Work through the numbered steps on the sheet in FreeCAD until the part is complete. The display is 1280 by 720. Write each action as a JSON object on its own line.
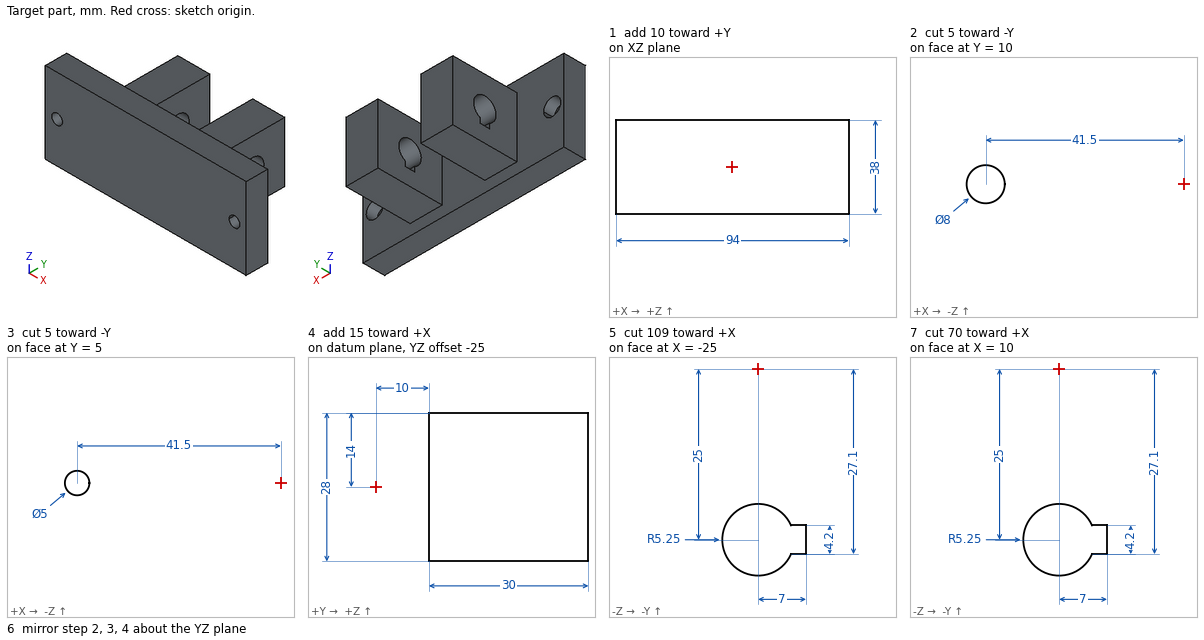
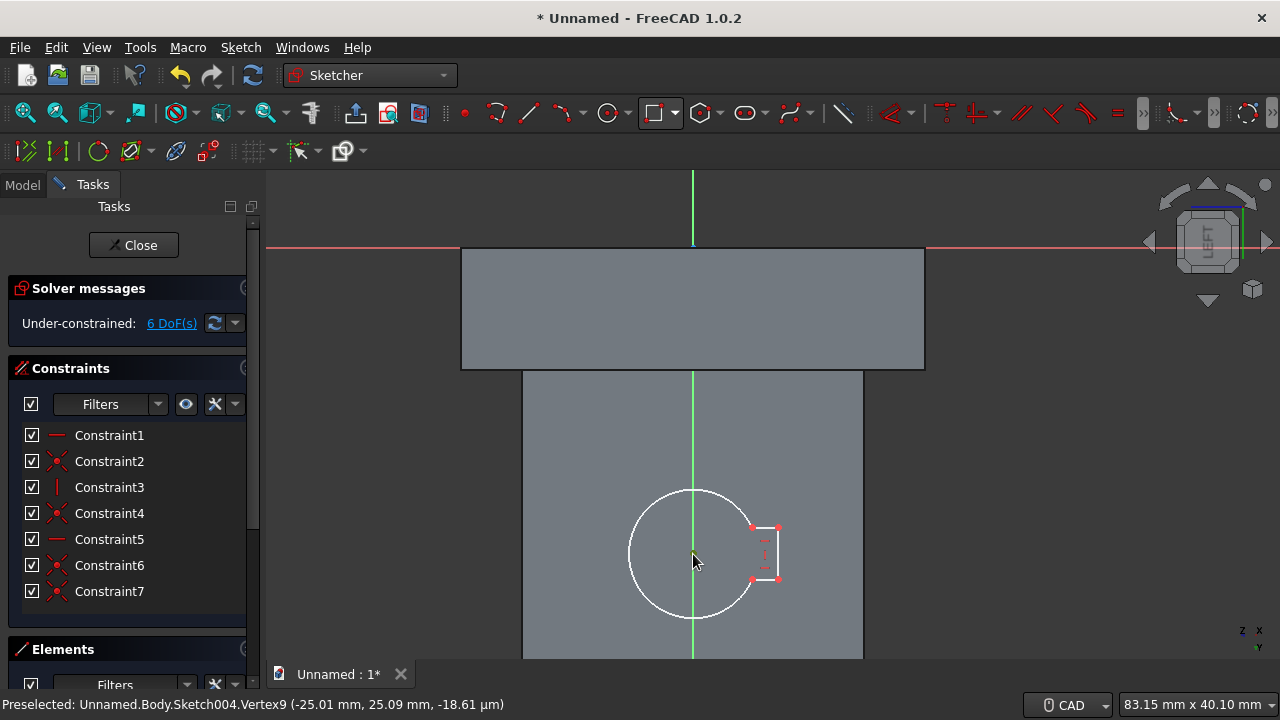
{"action": "left_click", "coordinate": [693, 569]}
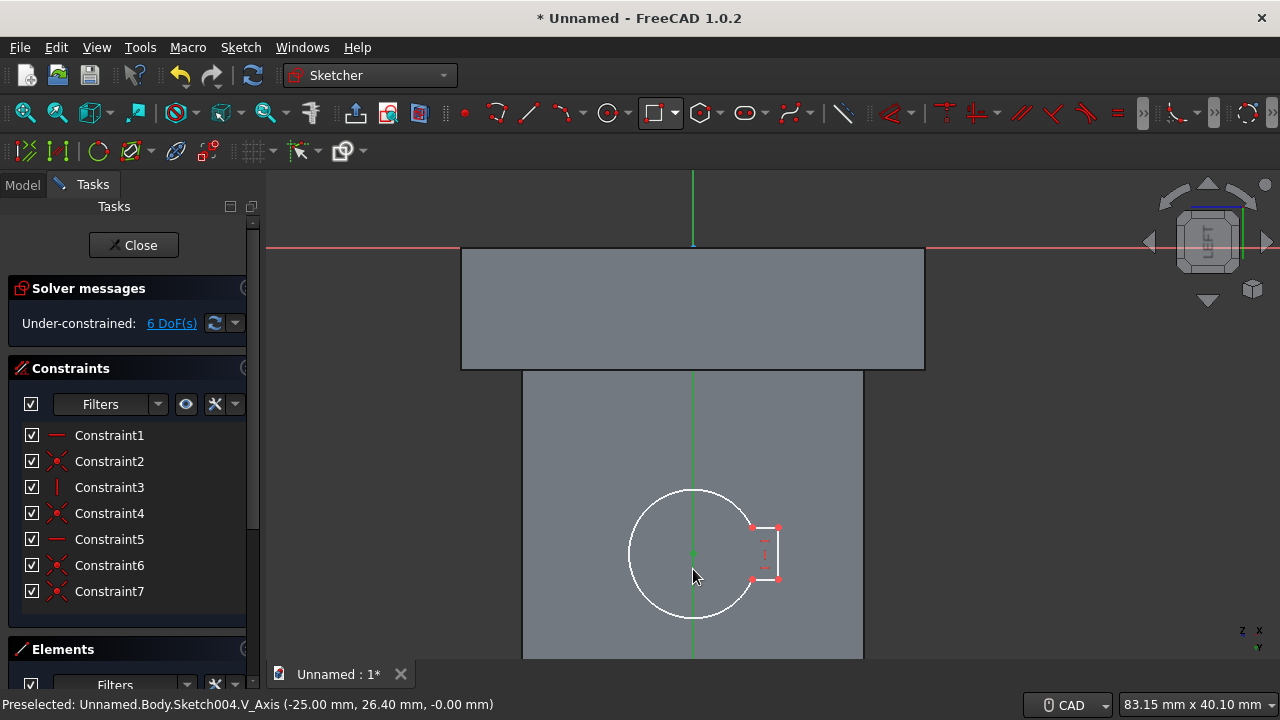
{"action": "left_click", "coordinate": [946, 114]}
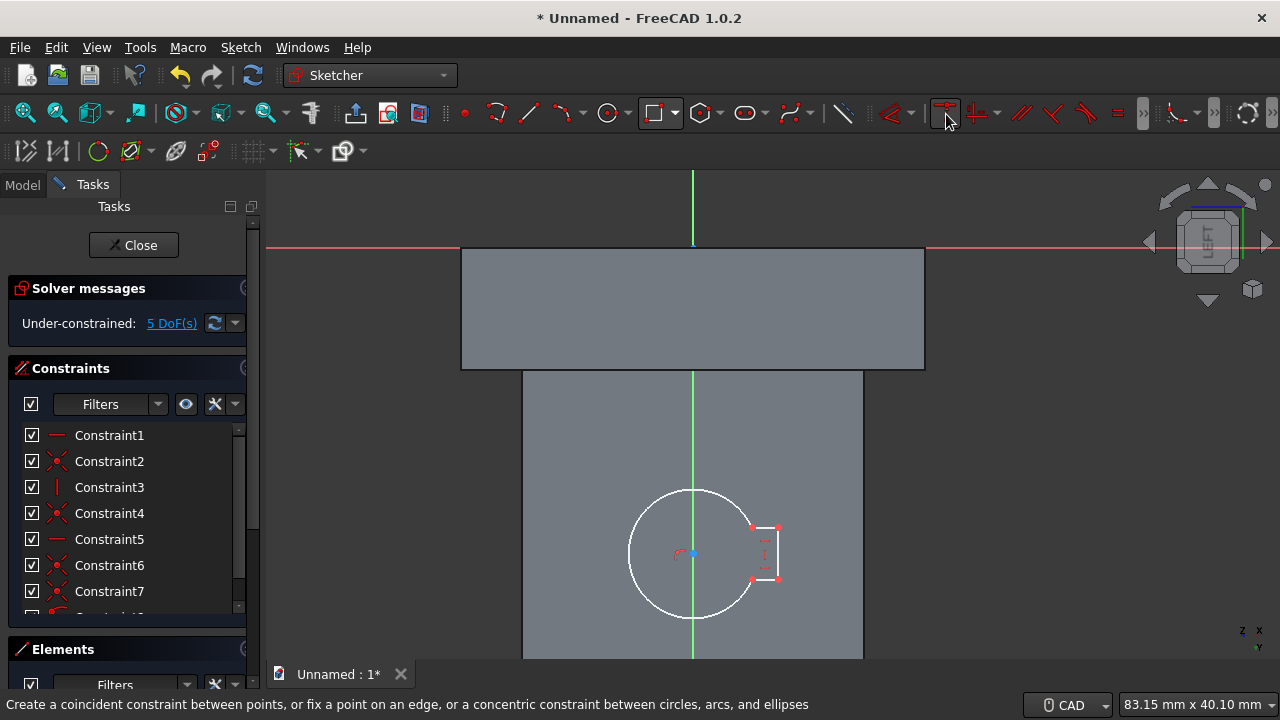
{"action": "left_click", "coordinate": [890, 114]}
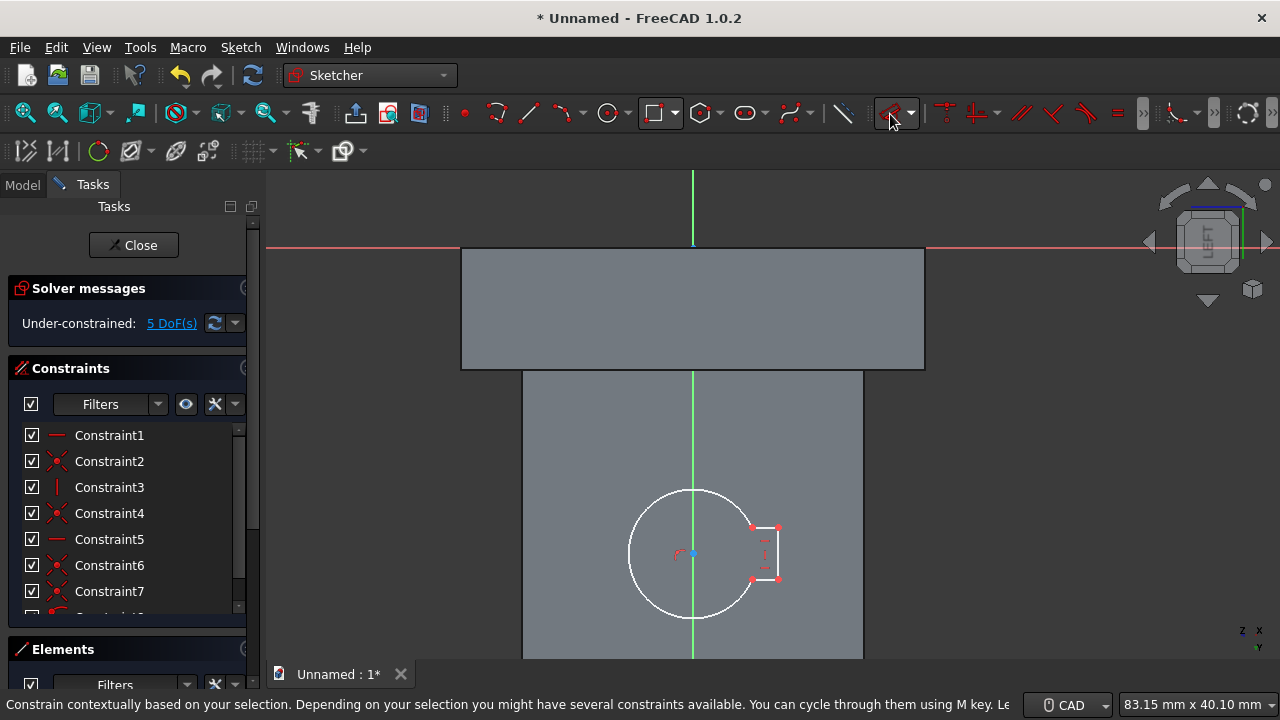
{"action": "left_click", "coordinate": [663, 497]}
{"action": "left_click", "coordinate": [648, 469]}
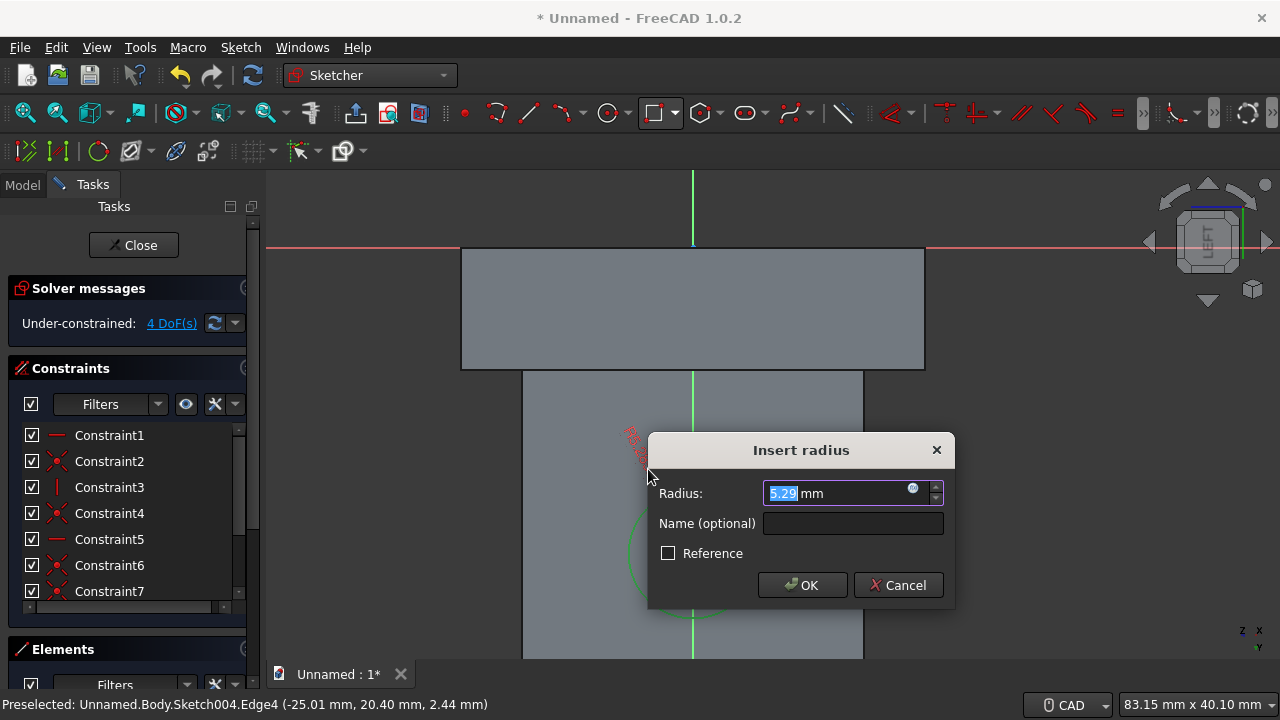
{"action": "type", "text": "5.25"}
{"action": "key", "text": "Return"}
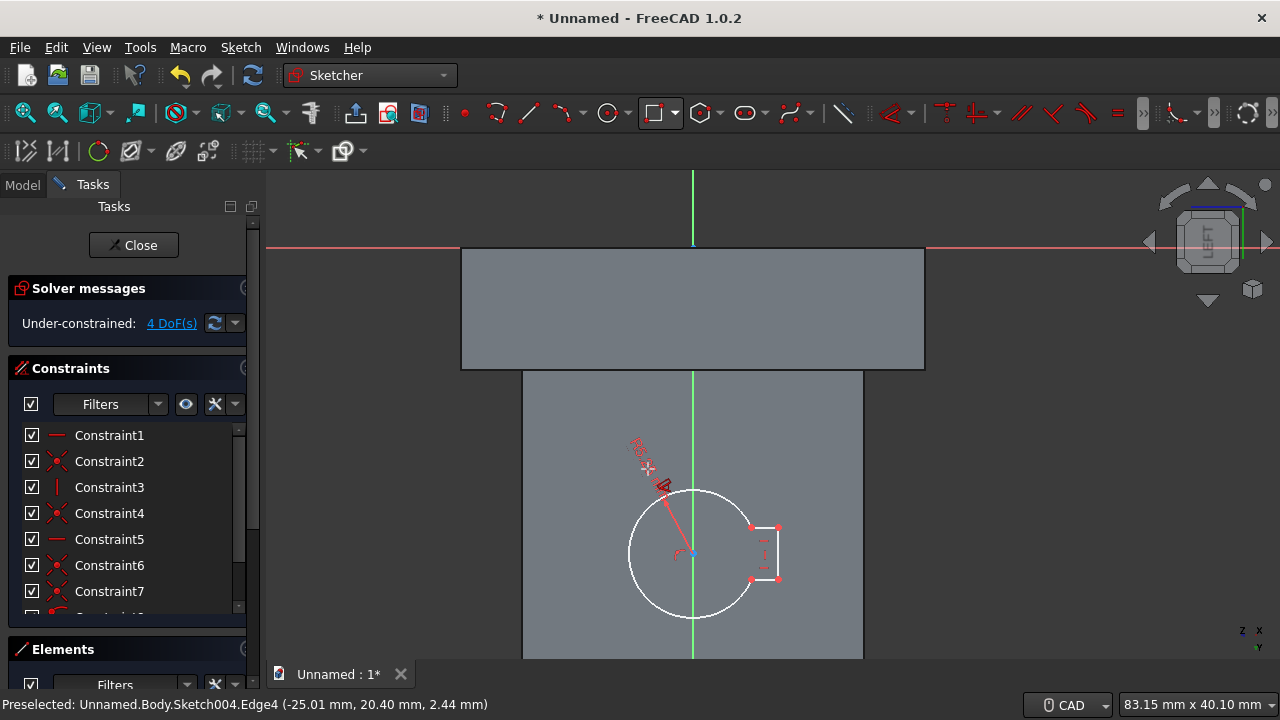
{"action": "left_click", "coordinate": [778, 580]}
{"action": "left_click", "coordinate": [755, 614]}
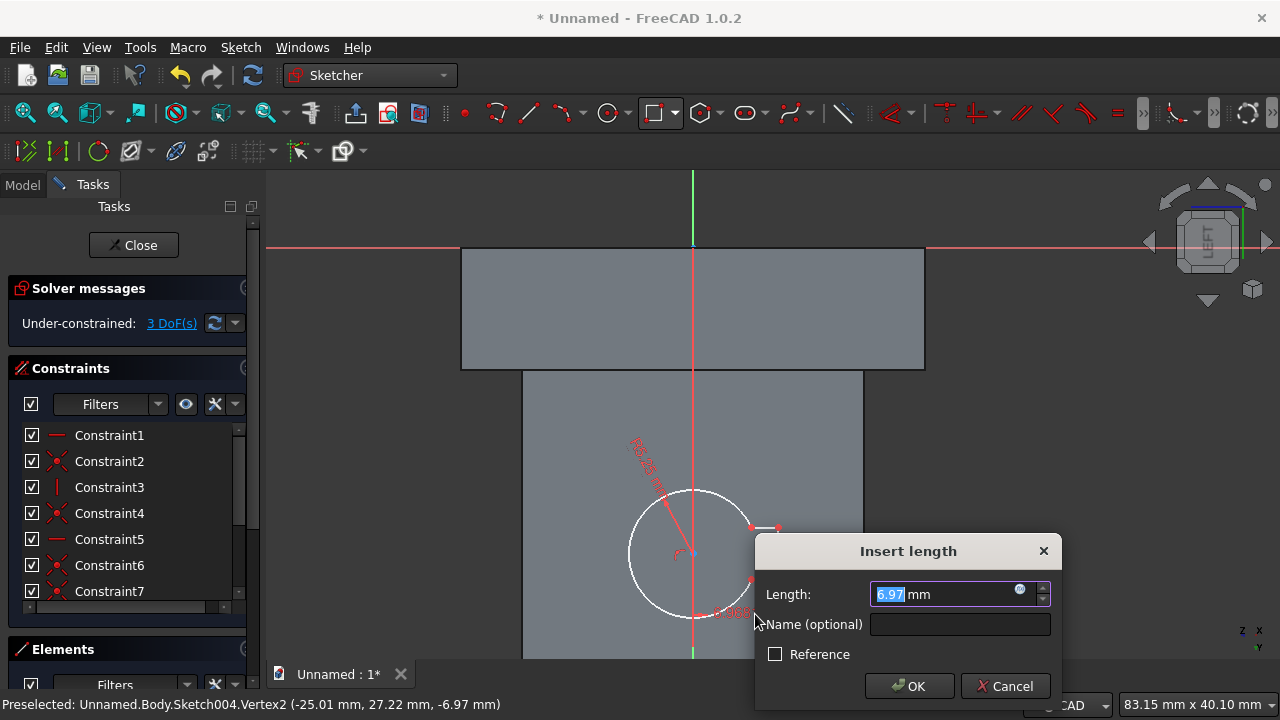
{"action": "type", "text": "7"}
{"action": "key", "text": "Return"}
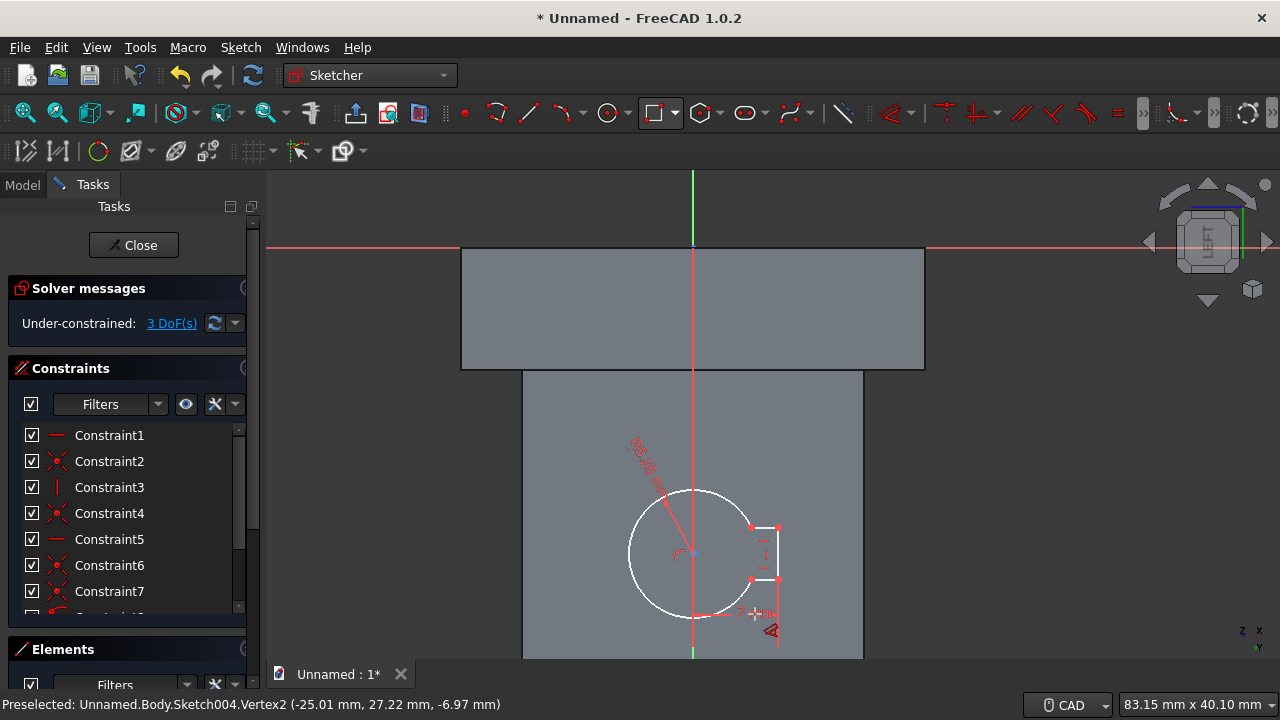
{"action": "left_click", "coordinate": [778, 564]}
{"action": "left_click", "coordinate": [812, 554]}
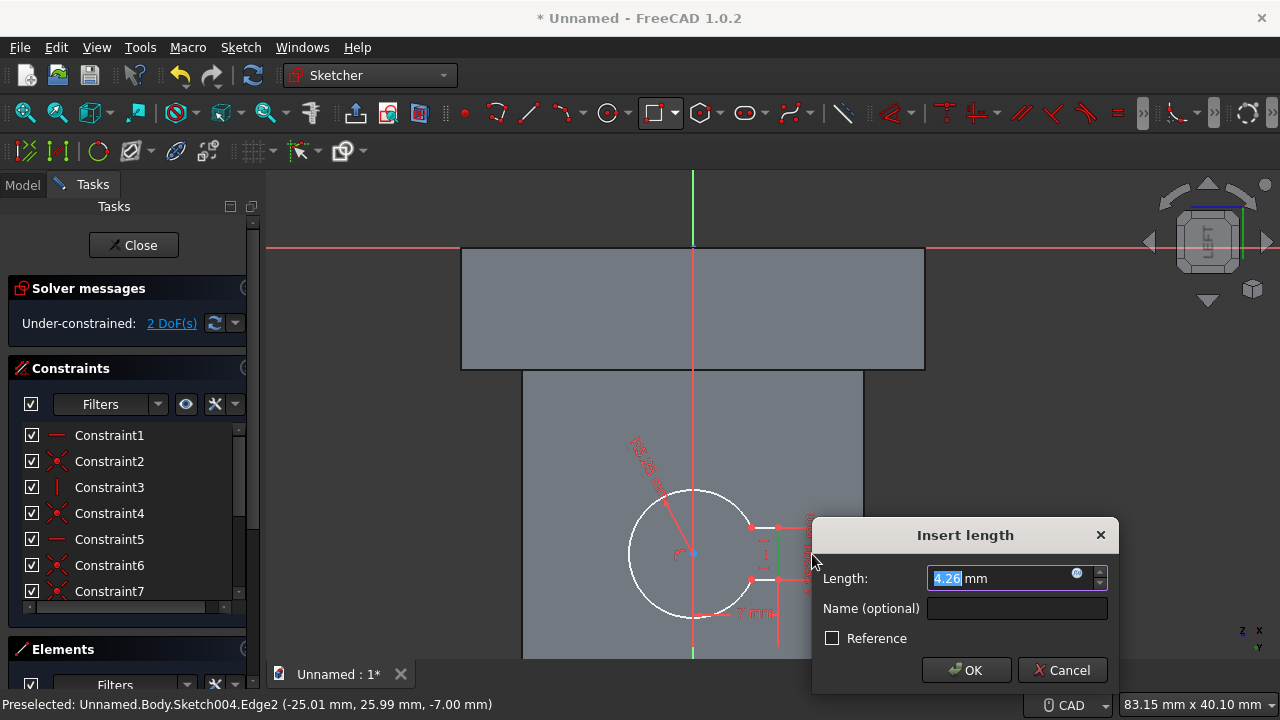
{"action": "type", "text": "4.2"}
{"action": "key", "text": "Return"}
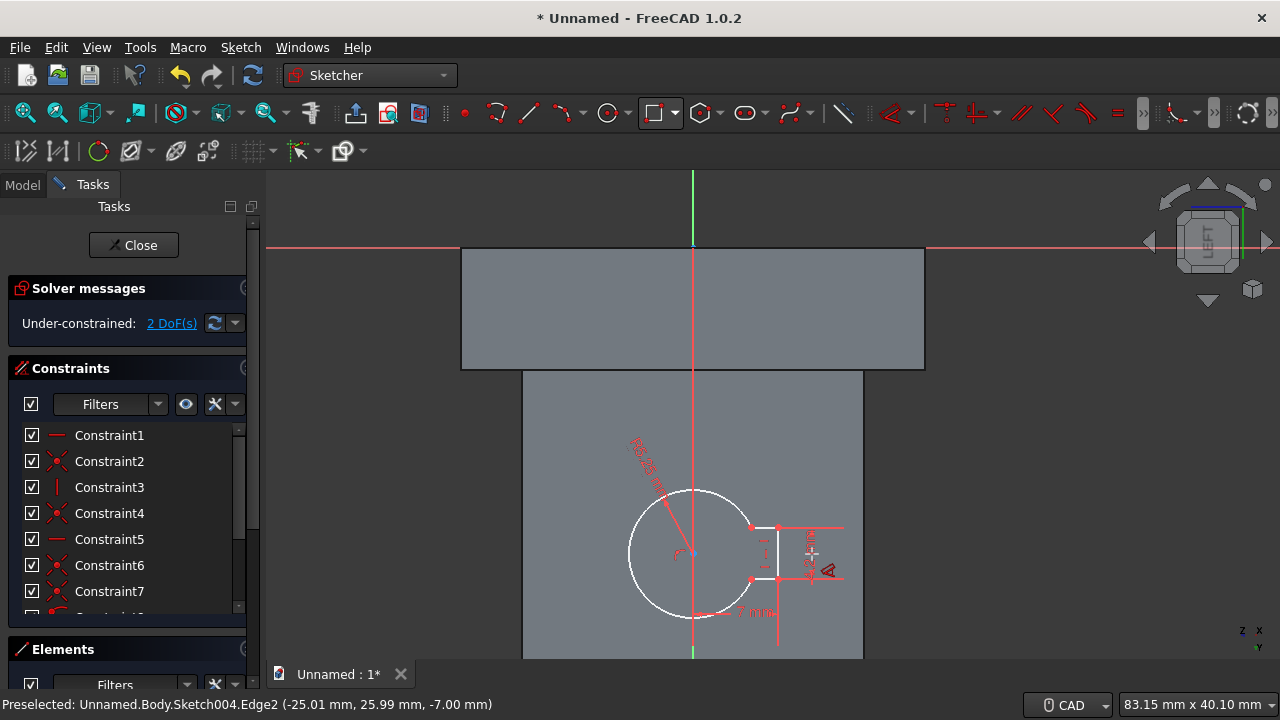
{"action": "left_click", "coordinate": [693, 554]}
{"action": "left_click", "coordinate": [659, 401]}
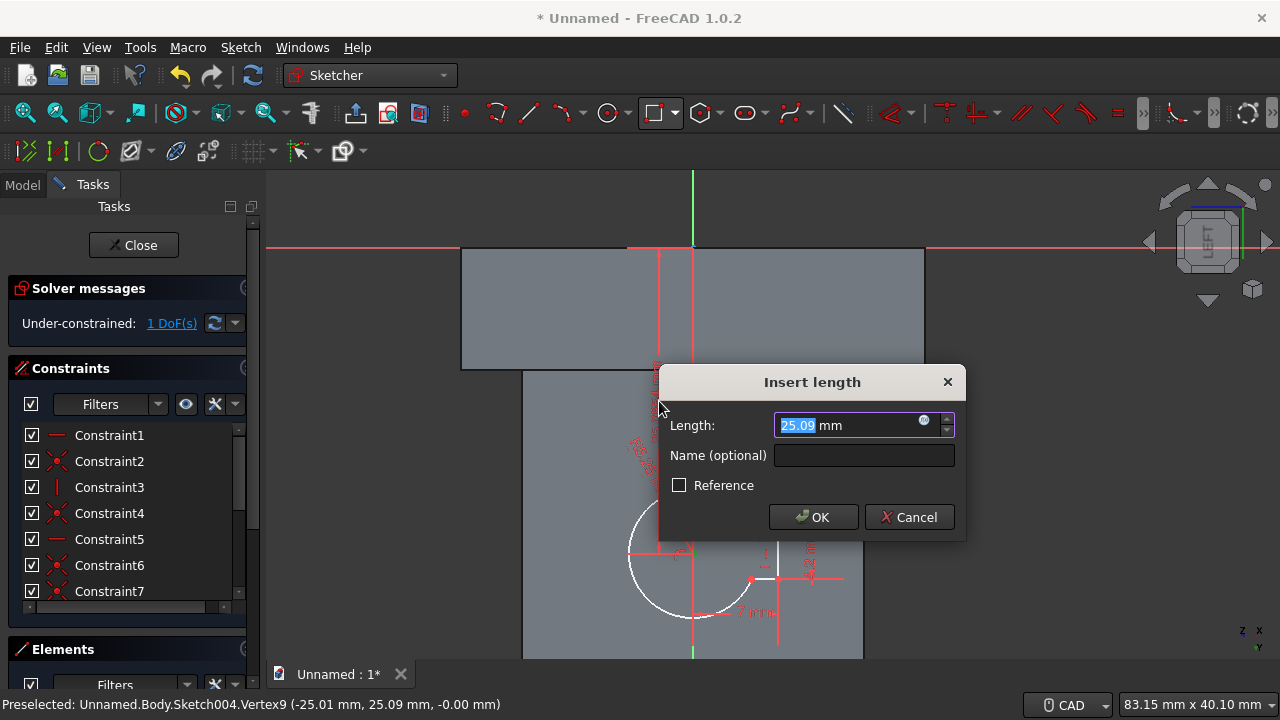
{"action": "type", "text": "25"}
{"action": "key", "text": "Return"}